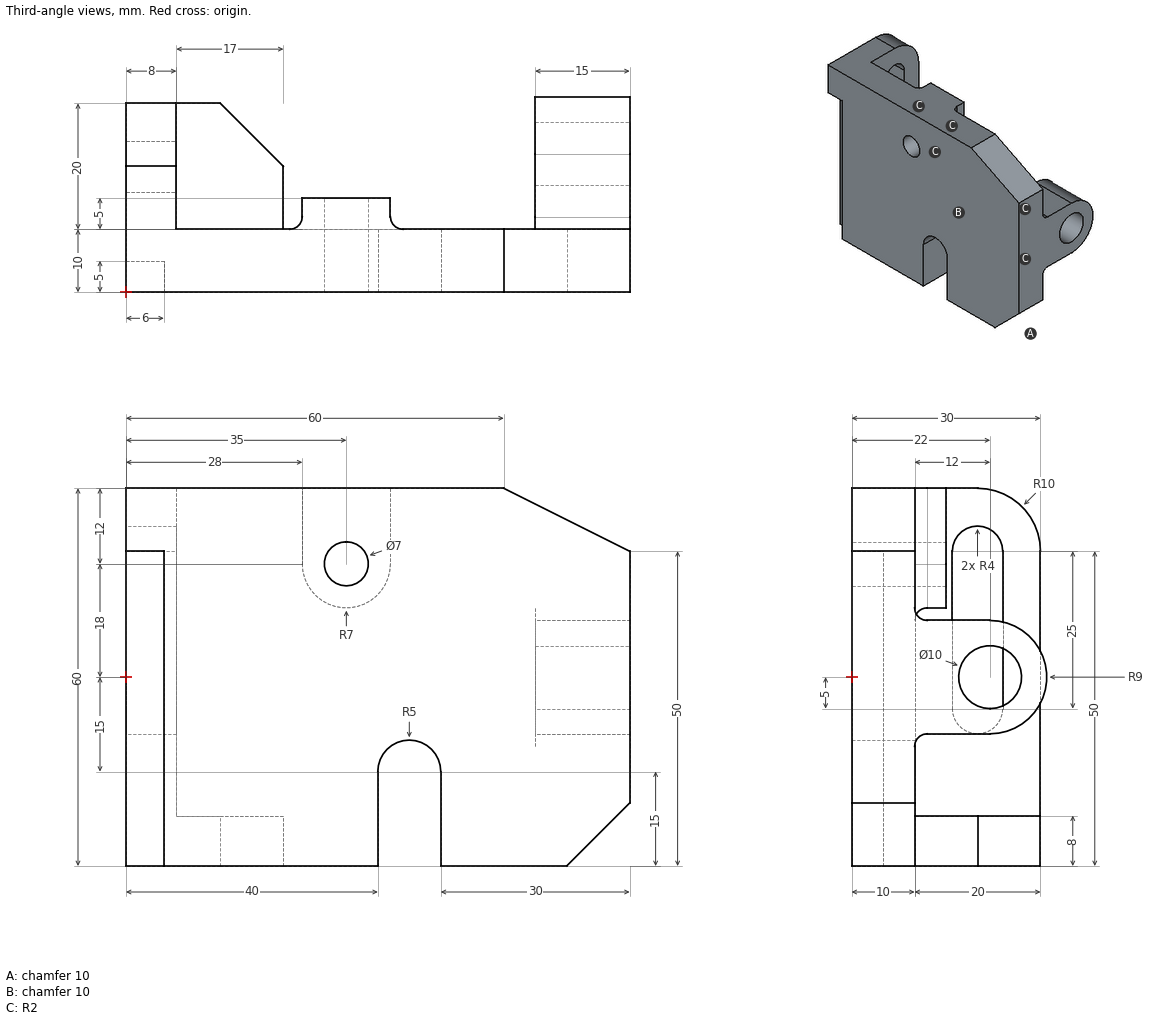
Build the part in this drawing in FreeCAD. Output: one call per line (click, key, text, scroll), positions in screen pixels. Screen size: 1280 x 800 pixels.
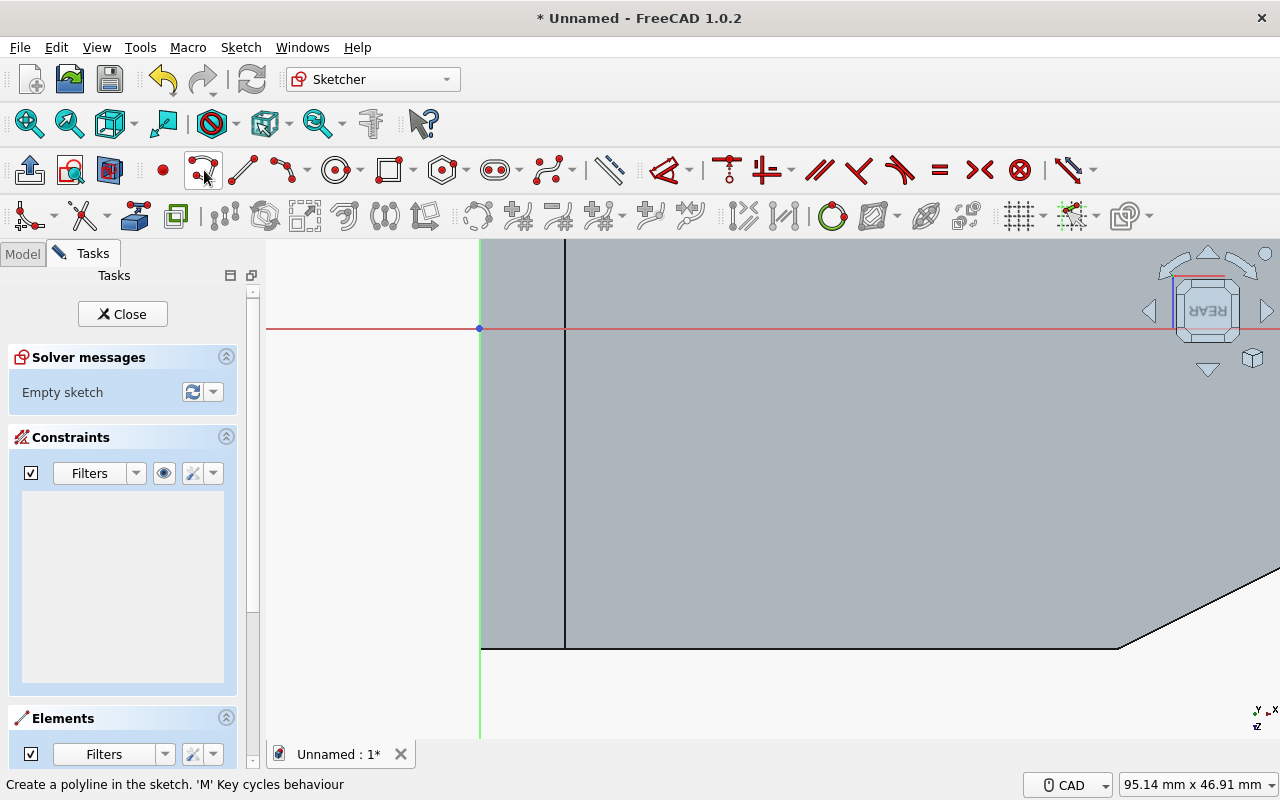
click(778, 521)
click(778, 648)
click(927, 648)
click(927, 521)
right_click(927, 521)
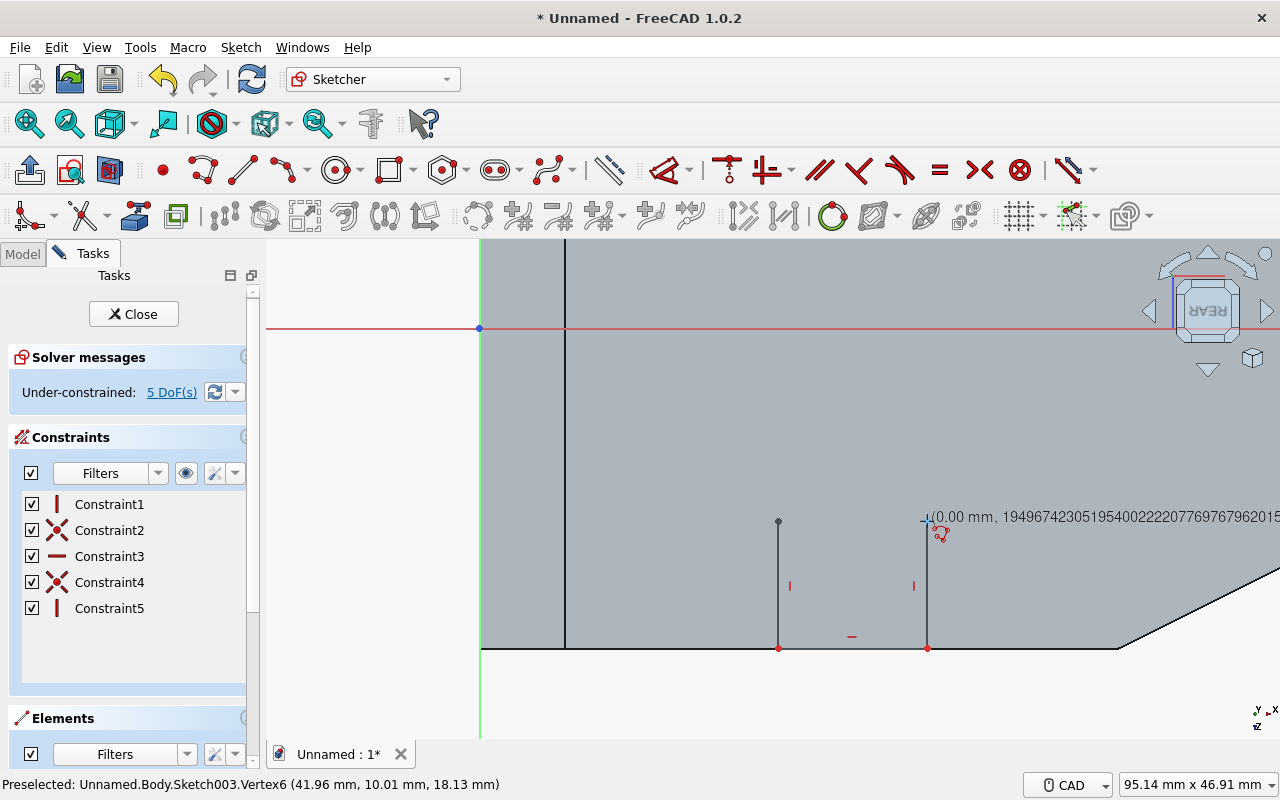
key(g)
key(3)
key(a)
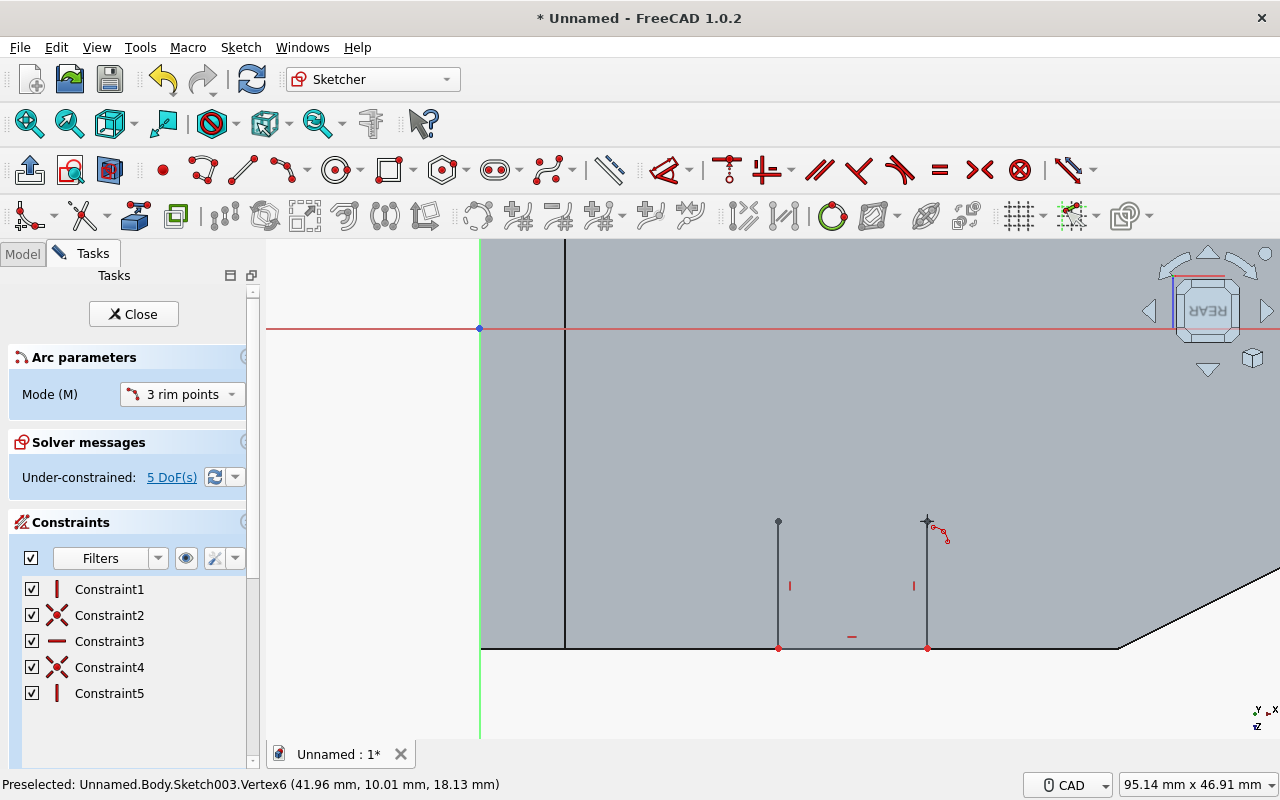
click(927, 522)
click(778, 522)
click(853, 446)
key(Escape)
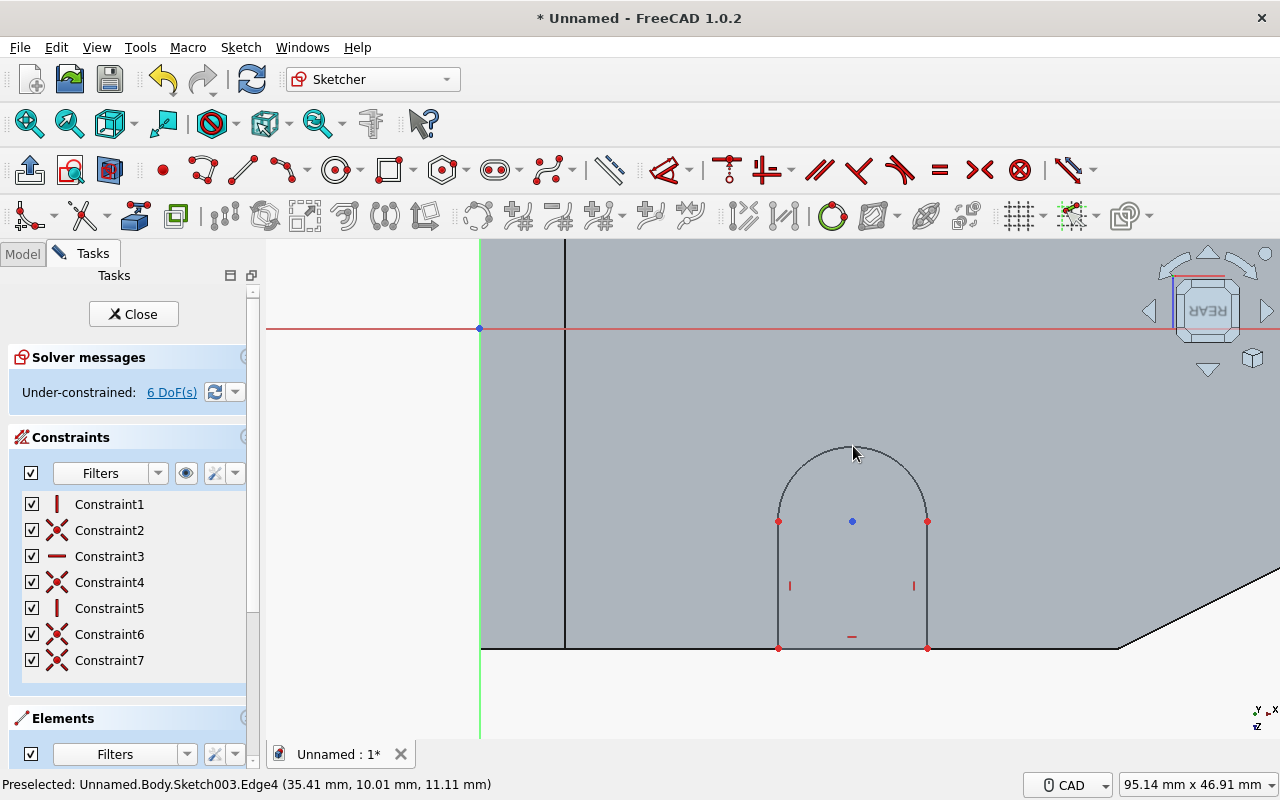
click(778, 560)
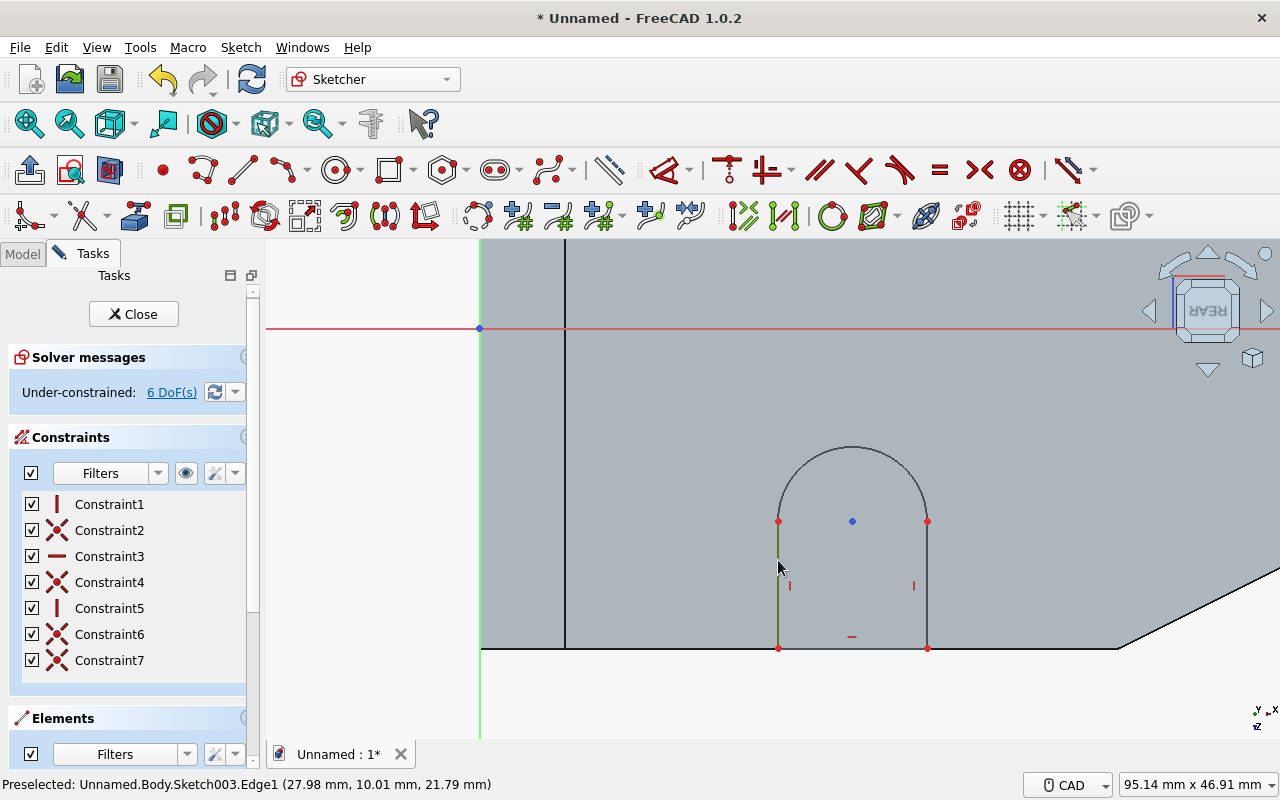
click(896, 461)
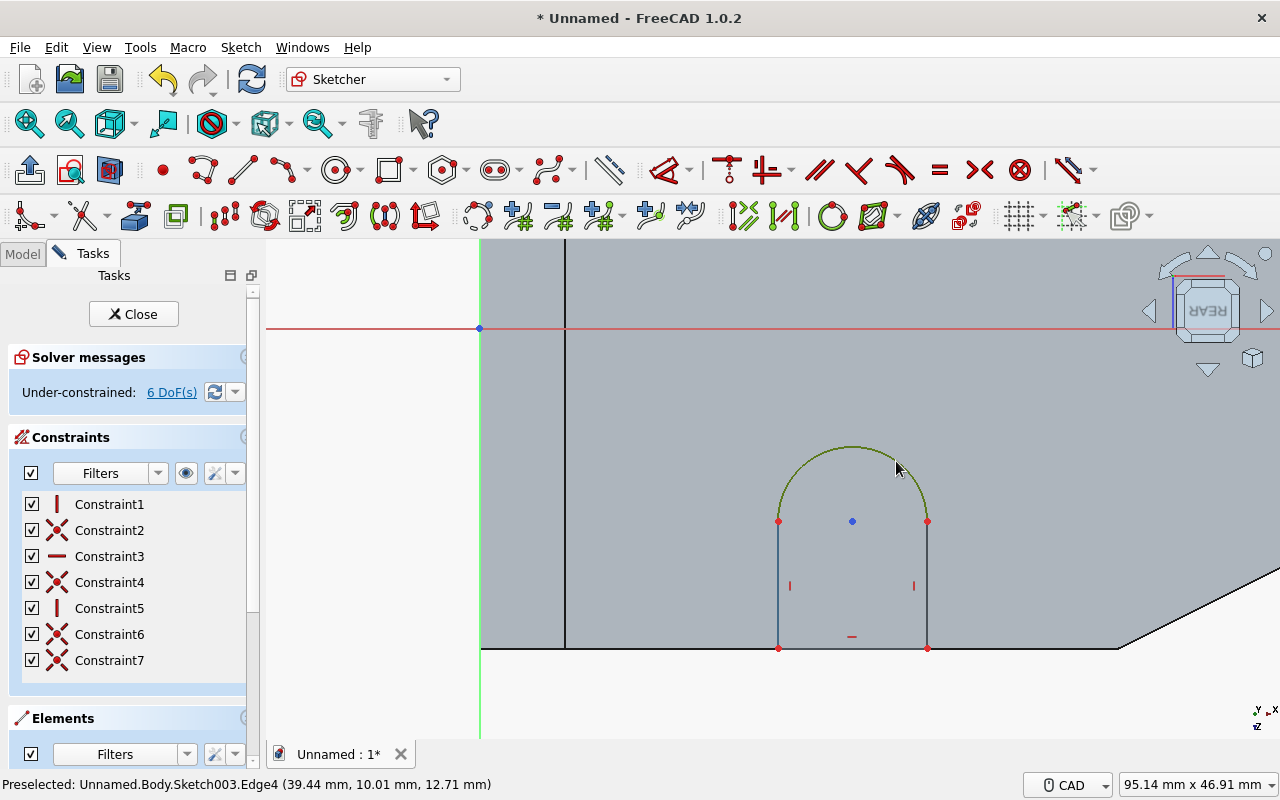
click(900, 170)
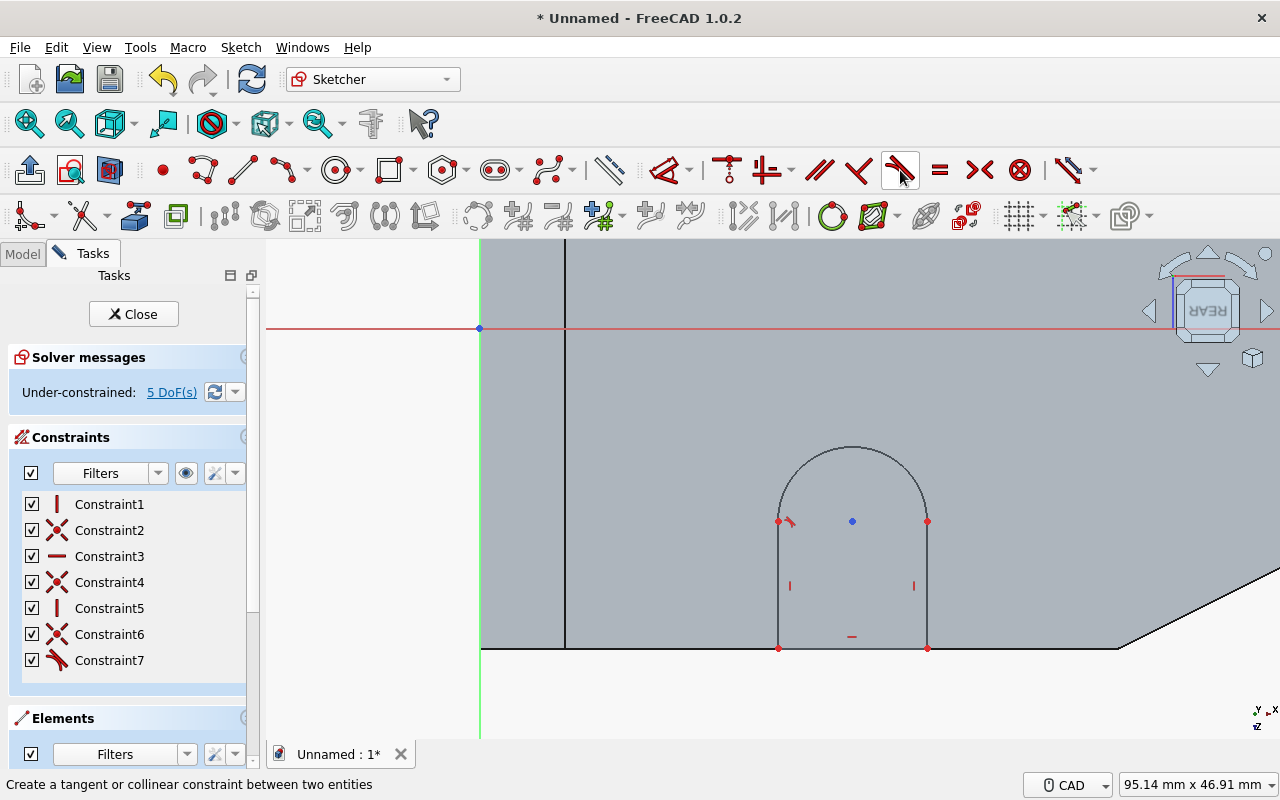
click(927, 611)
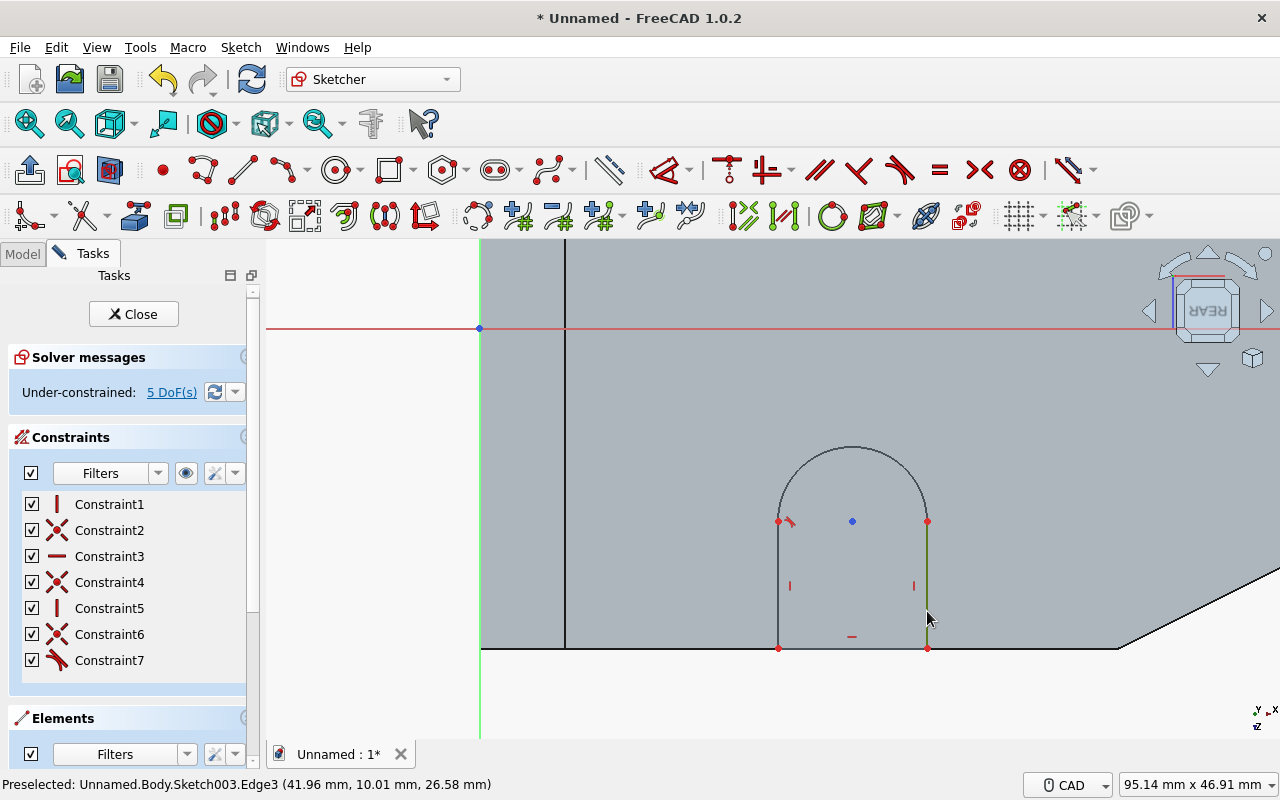
click(897, 461)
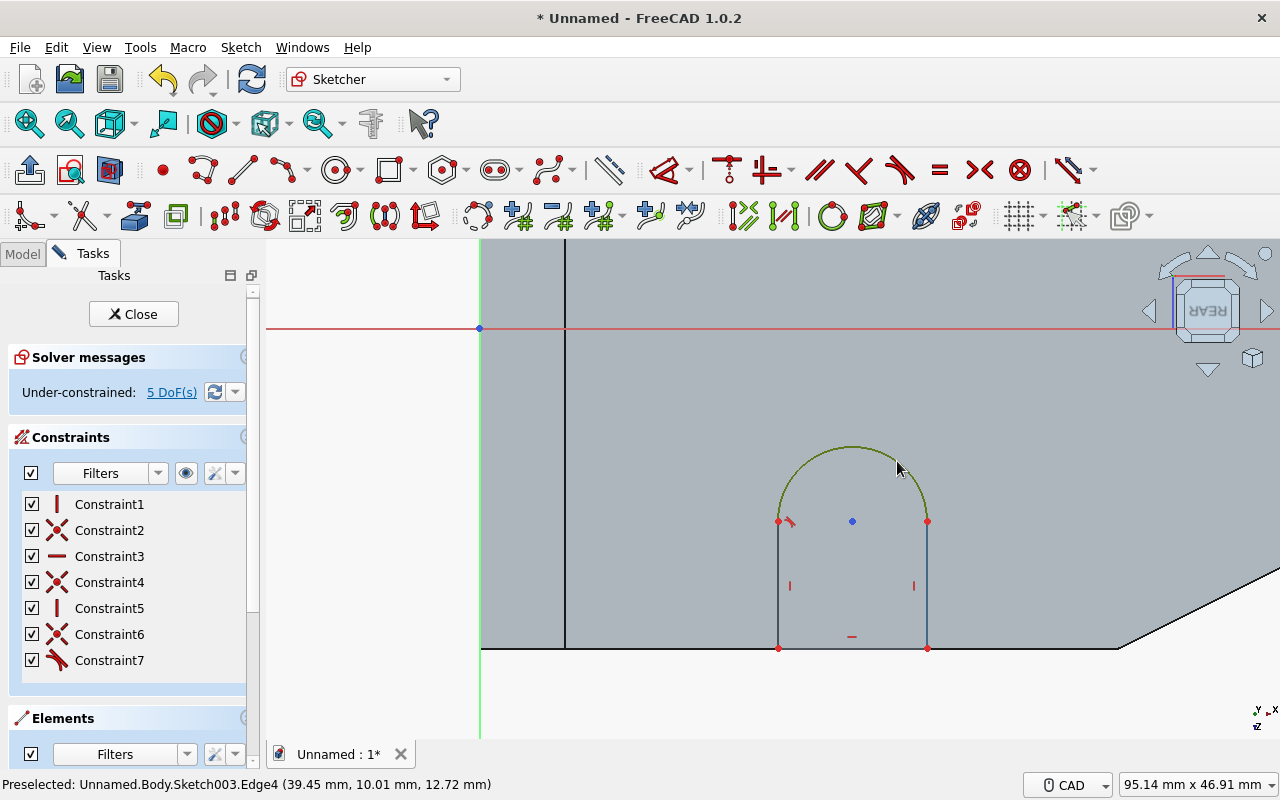
click(900, 170)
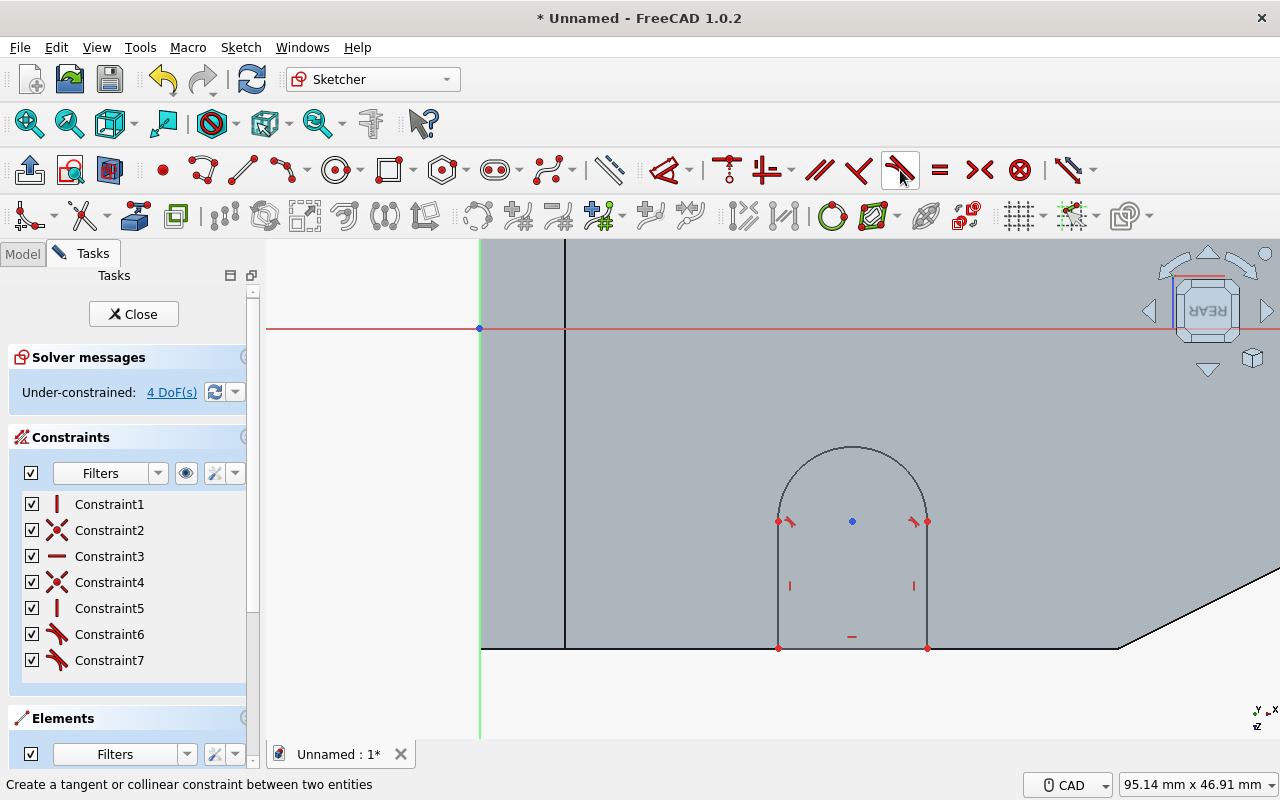
click(664, 170)